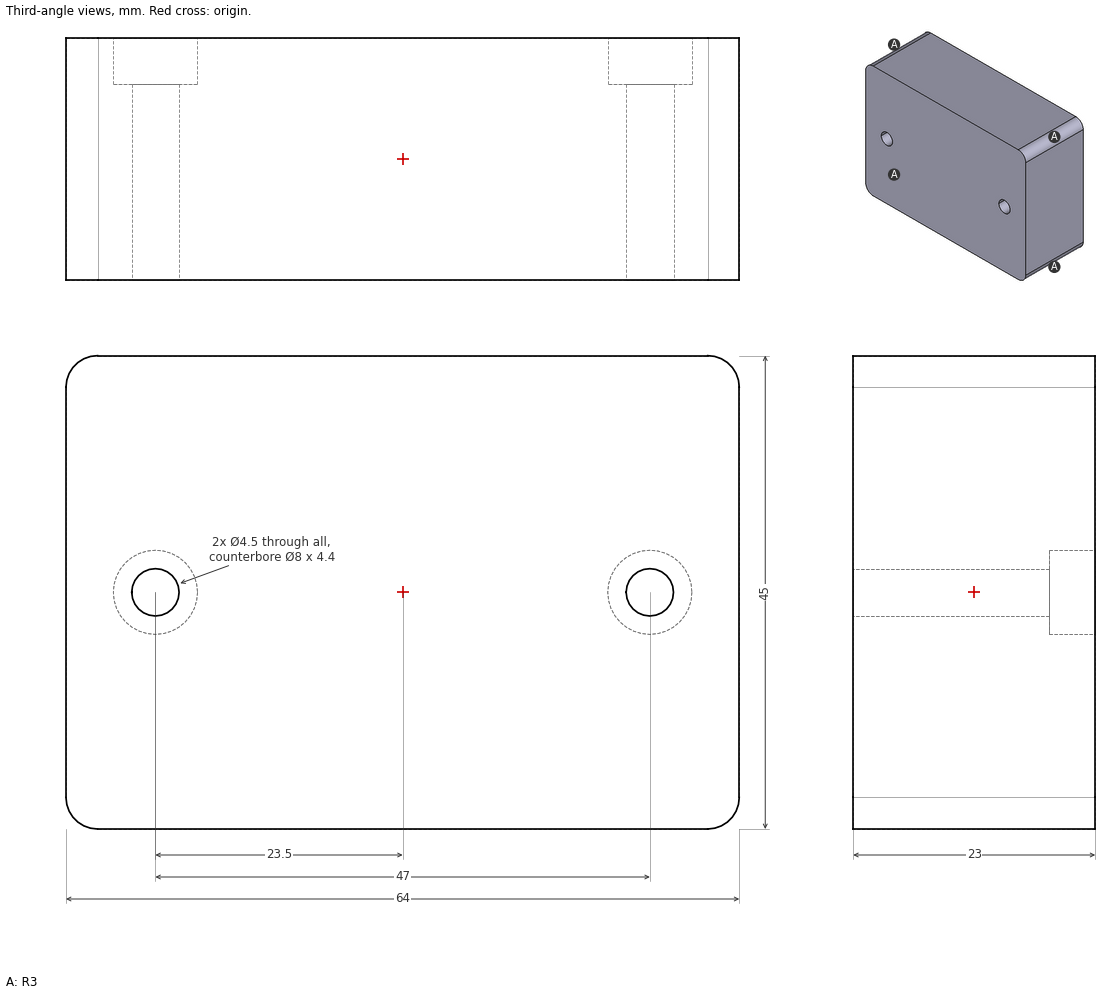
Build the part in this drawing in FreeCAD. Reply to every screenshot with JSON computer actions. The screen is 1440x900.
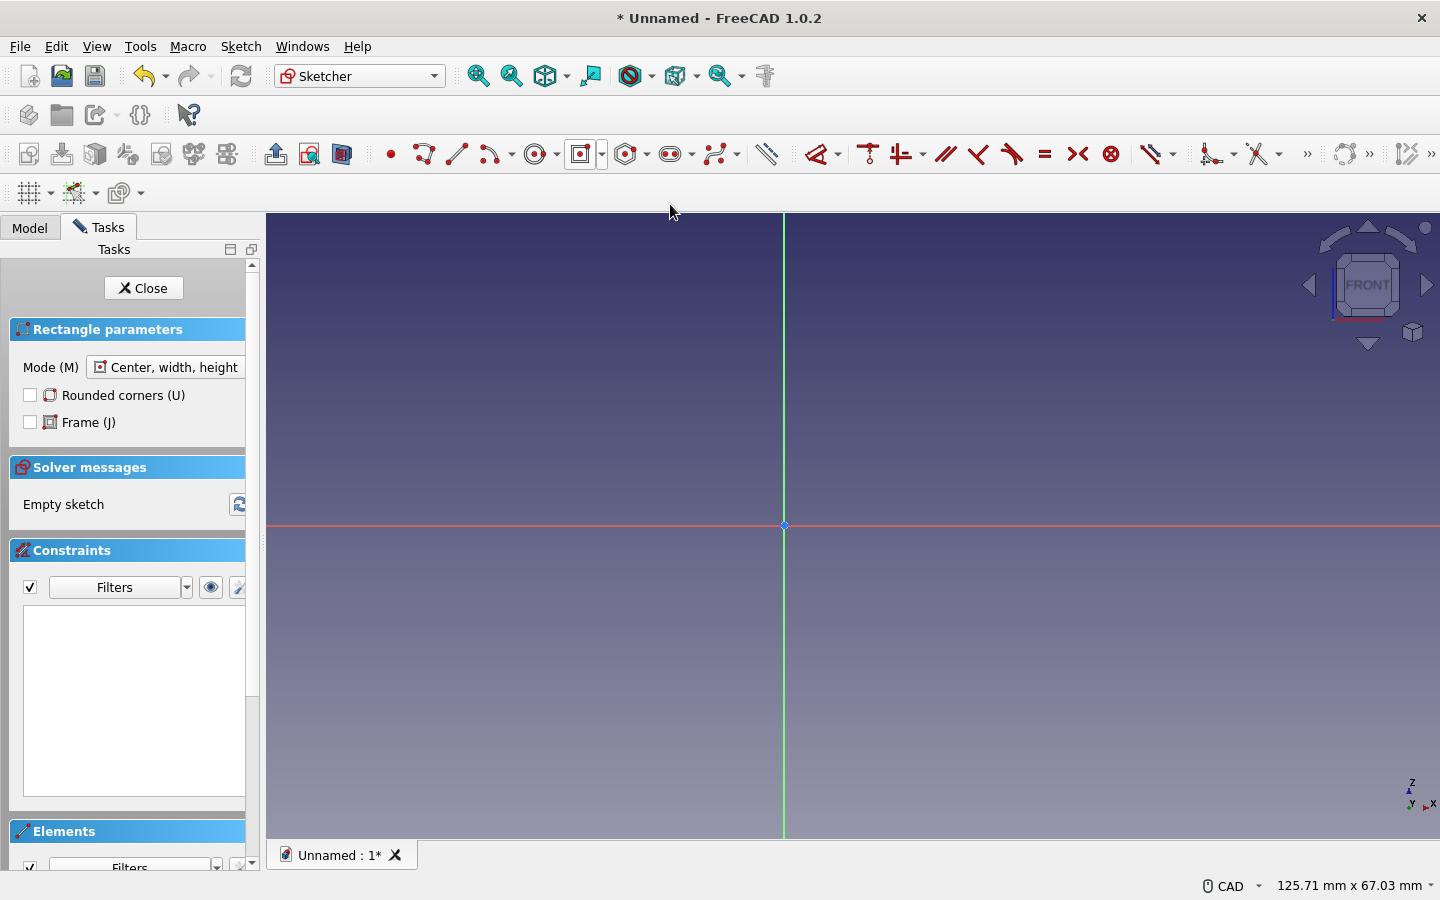
{"action": "left_click", "coordinate": [784, 526]}
{"action": "left_click", "coordinate": [1083, 316]}
{"action": "key", "text": "Escape"}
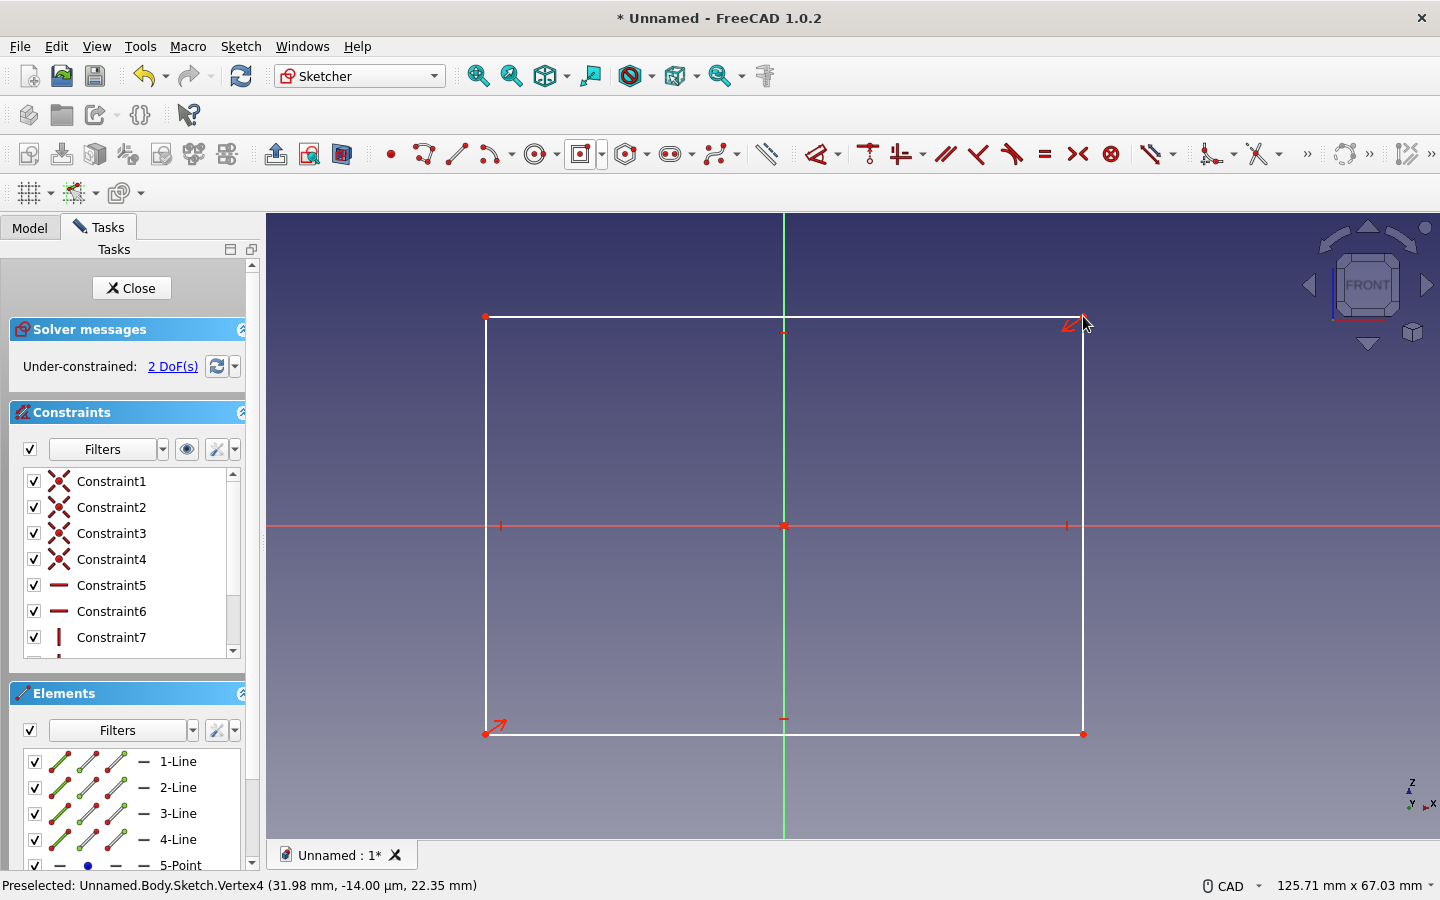
{"action": "left_click", "coordinate": [665, 735]}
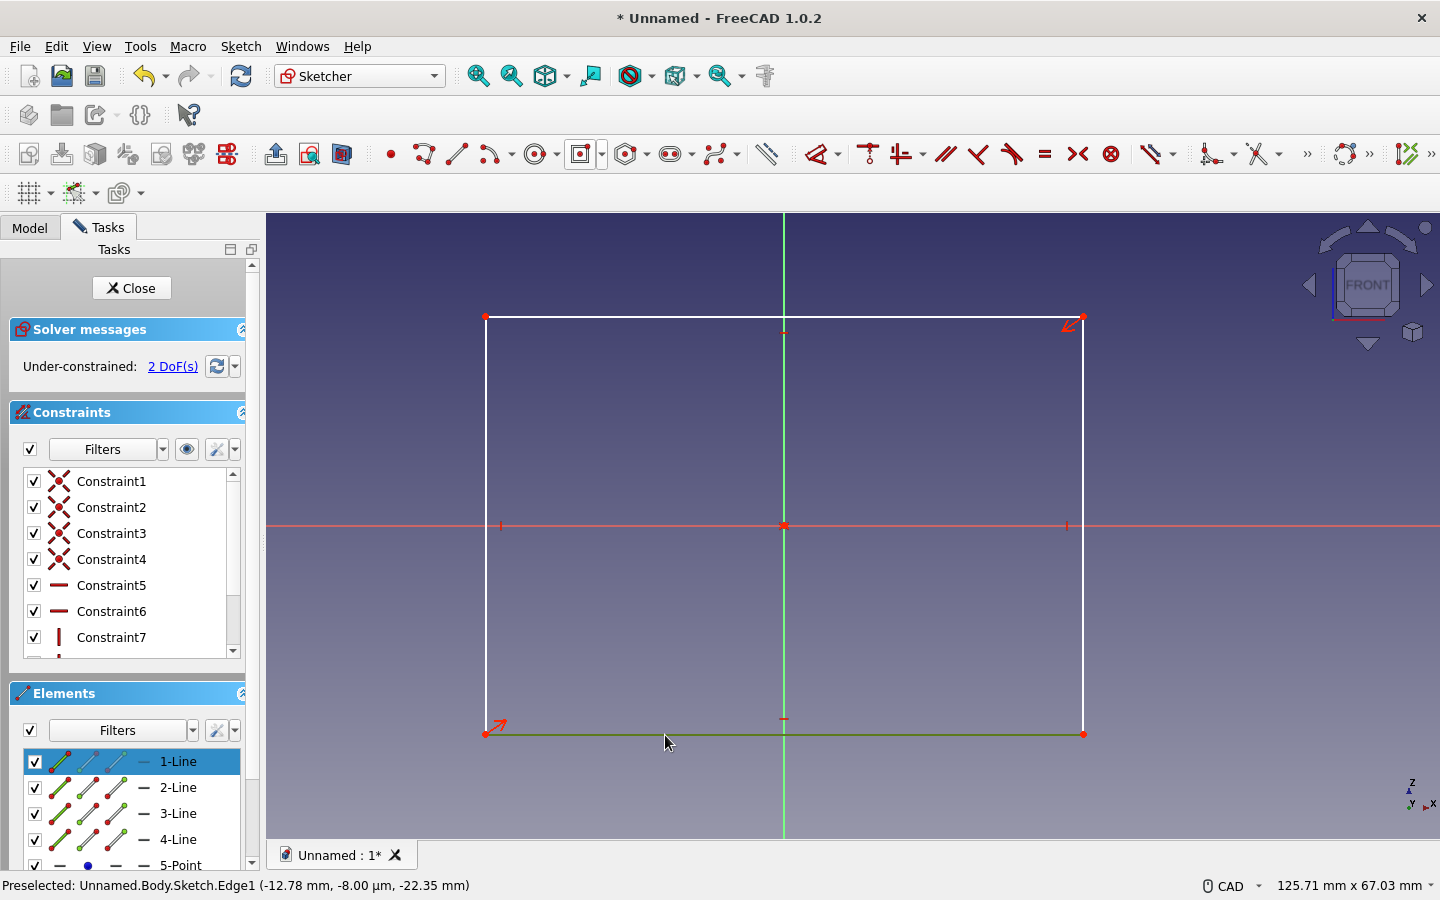
{"action": "key", "text": "l"}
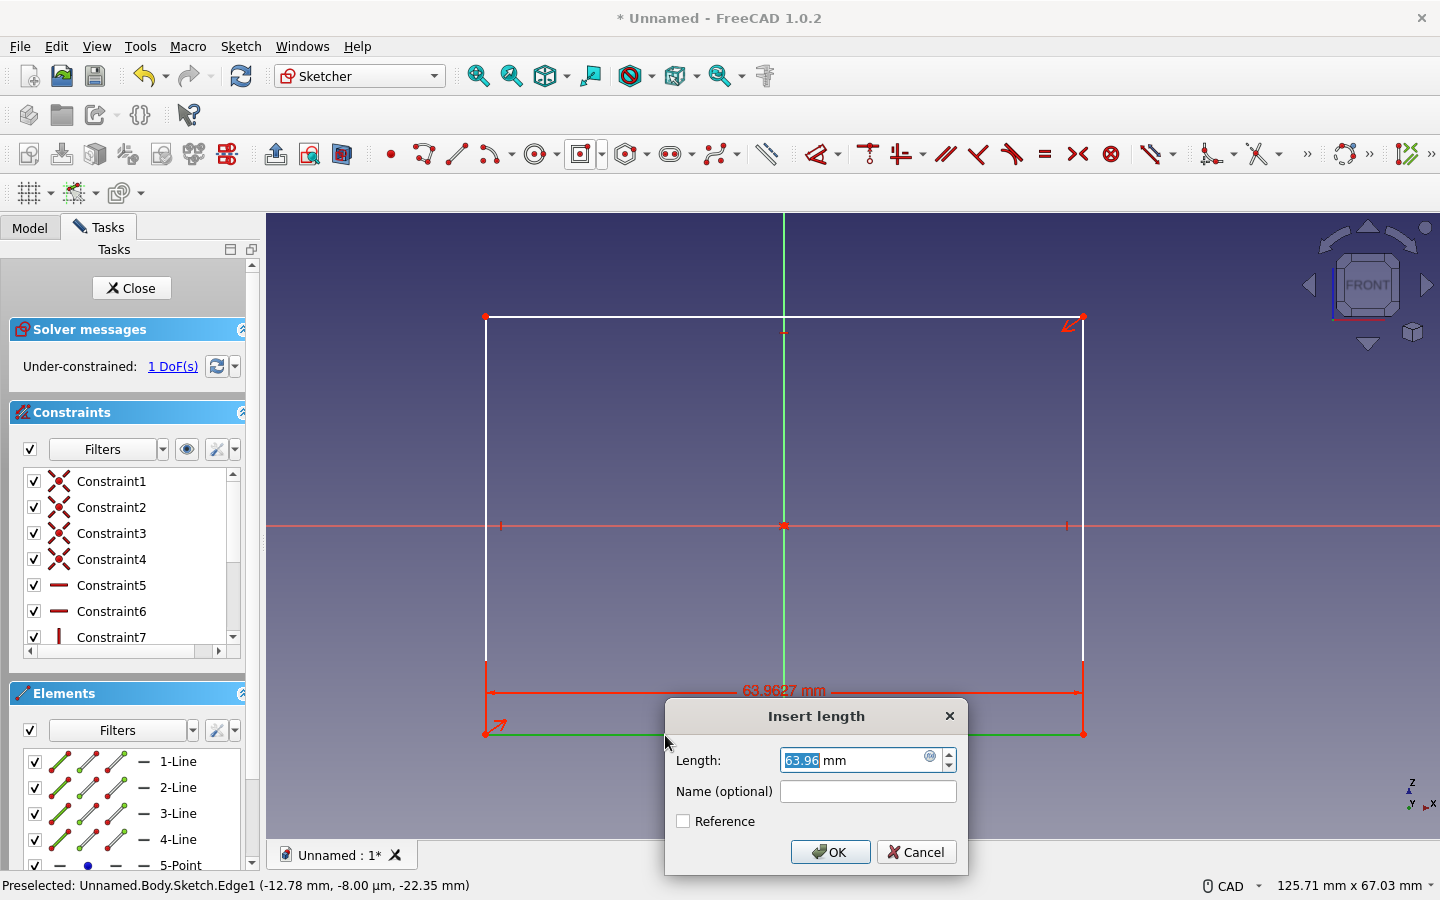
{"action": "type", "text": "64"}
{"action": "key", "text": "Return"}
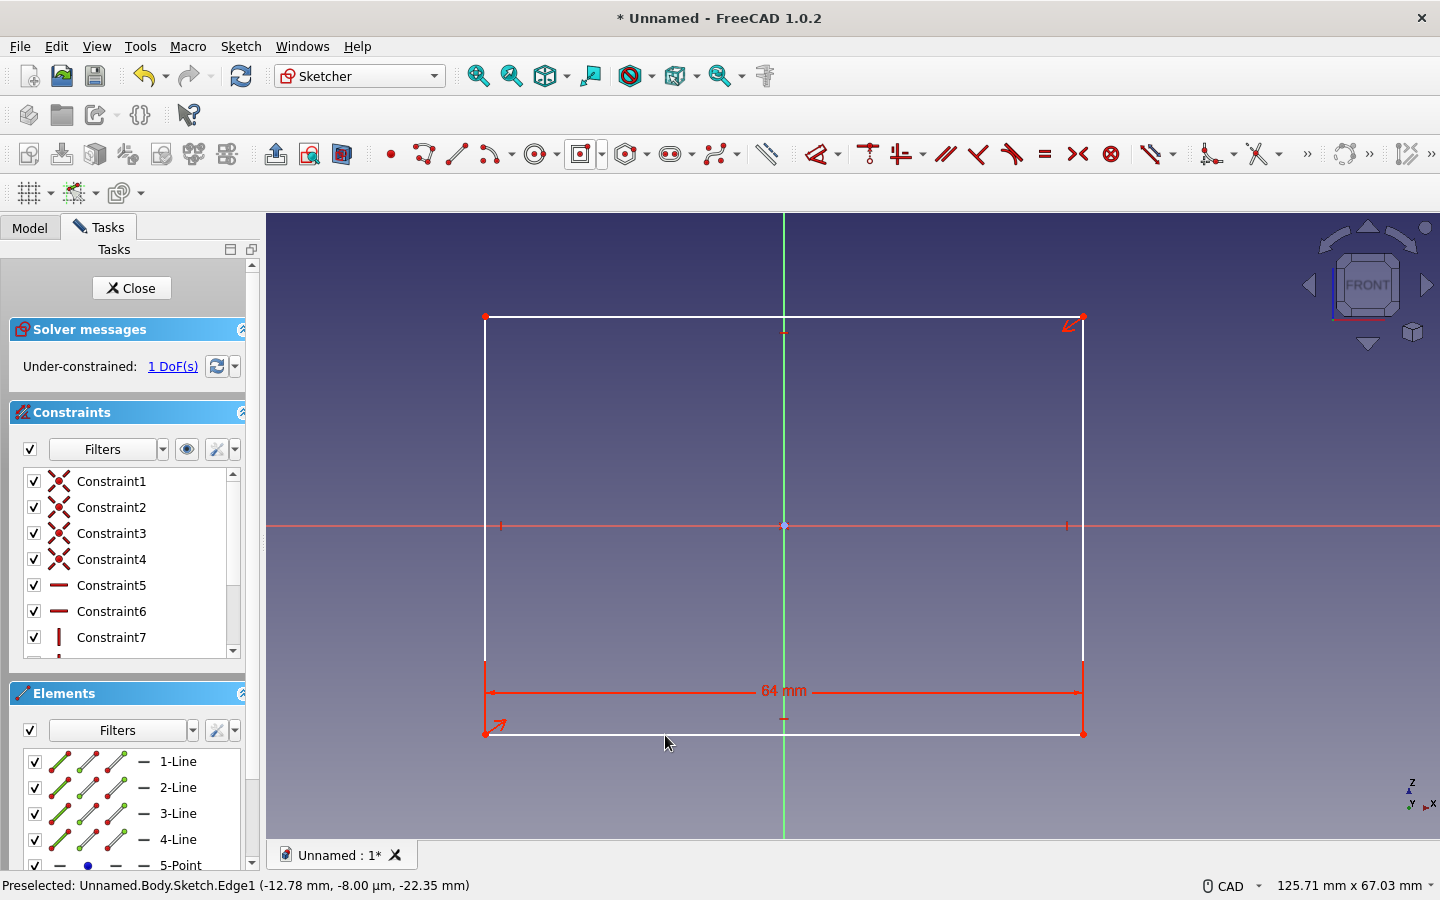
{"action": "left_click", "coordinate": [1083, 609]}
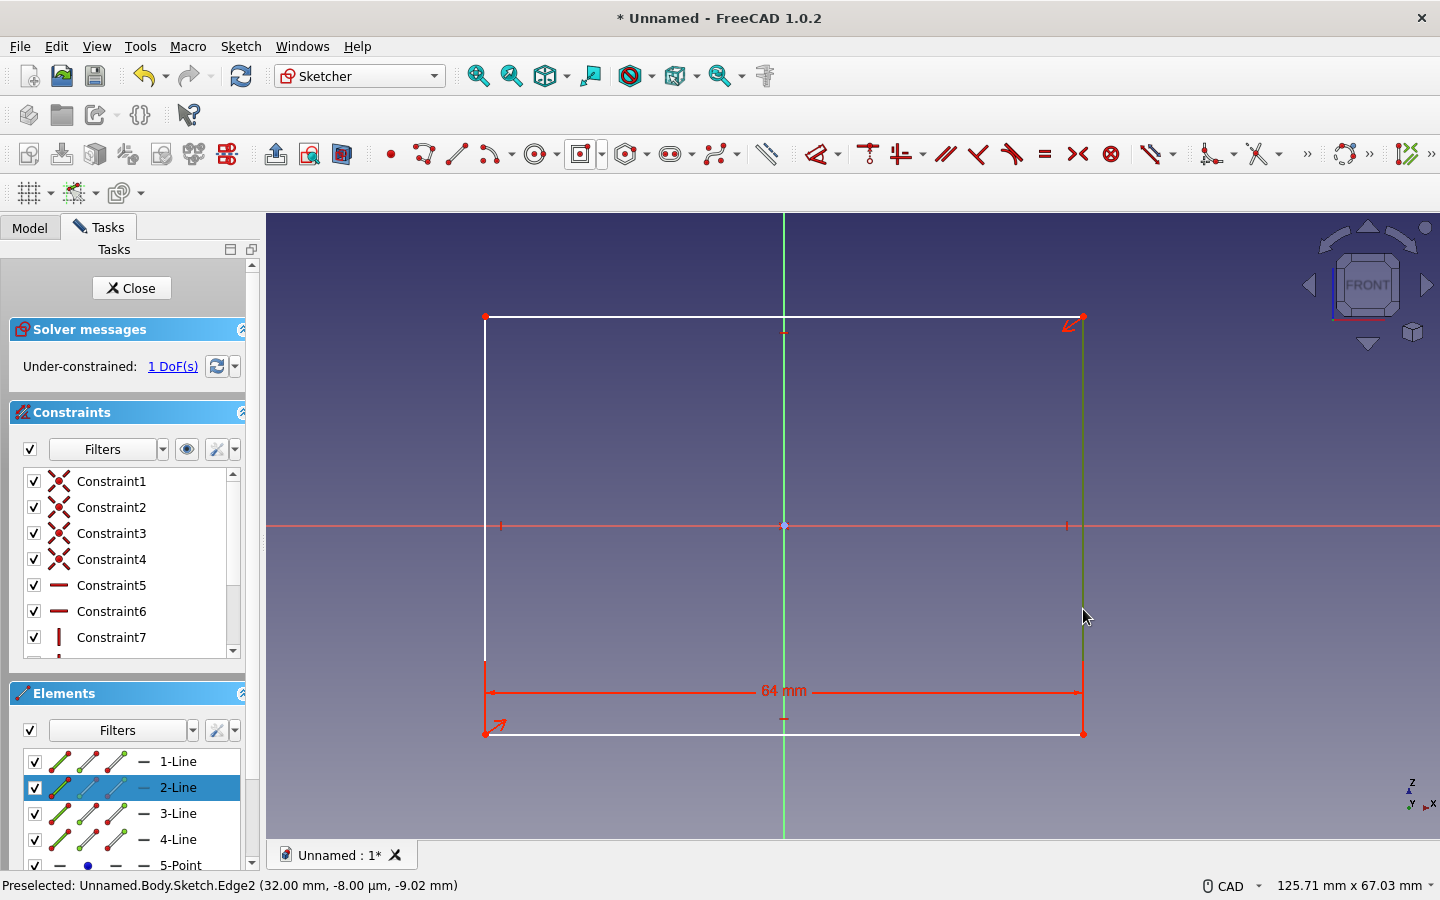
{"action": "key", "text": "i"}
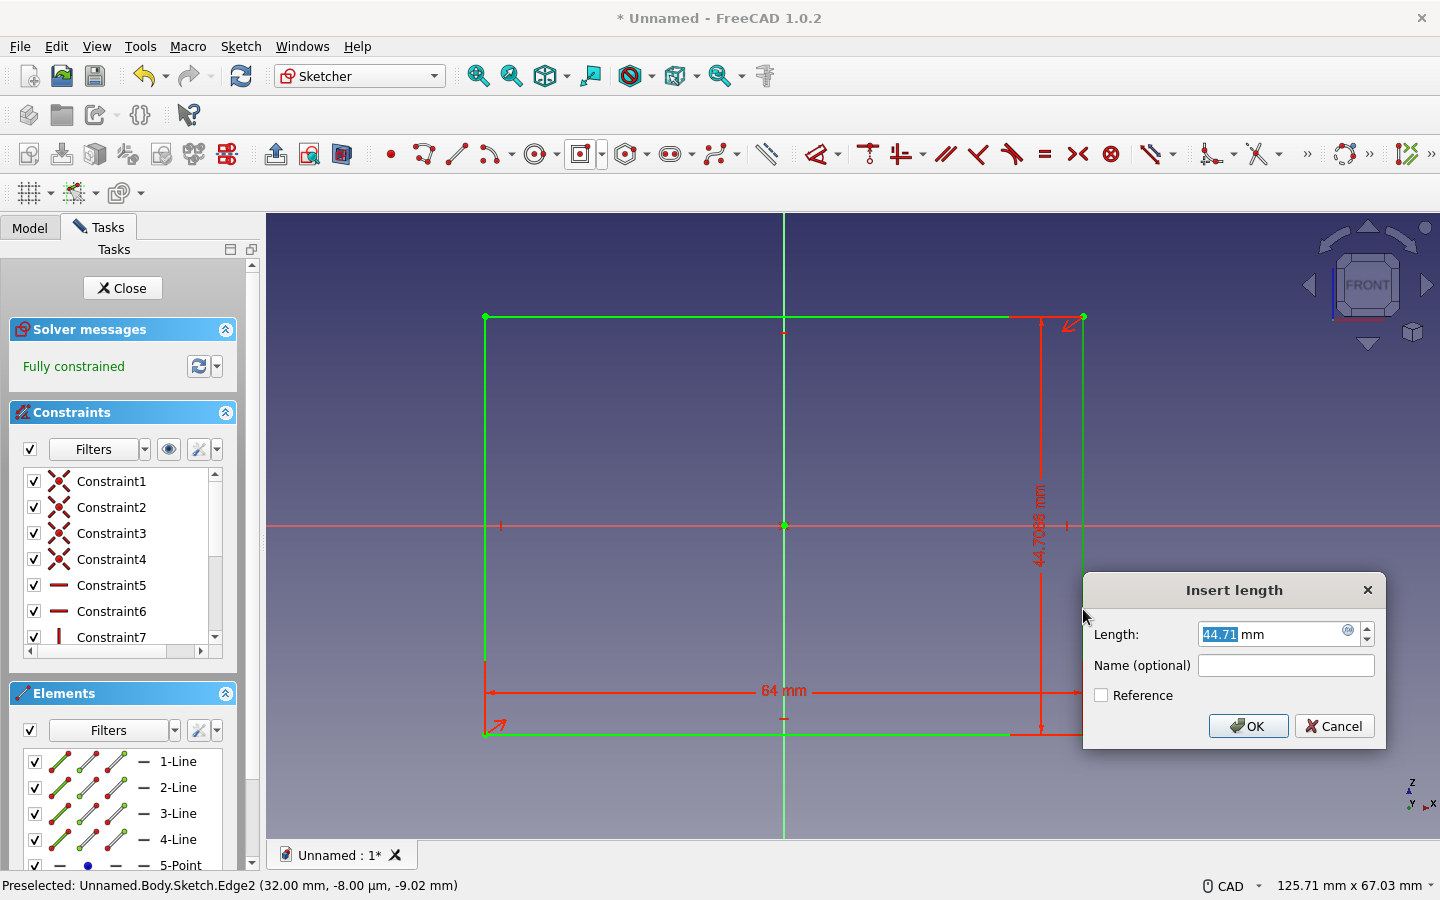
{"action": "type", "text": "45"}
{"action": "key", "text": "Return"}